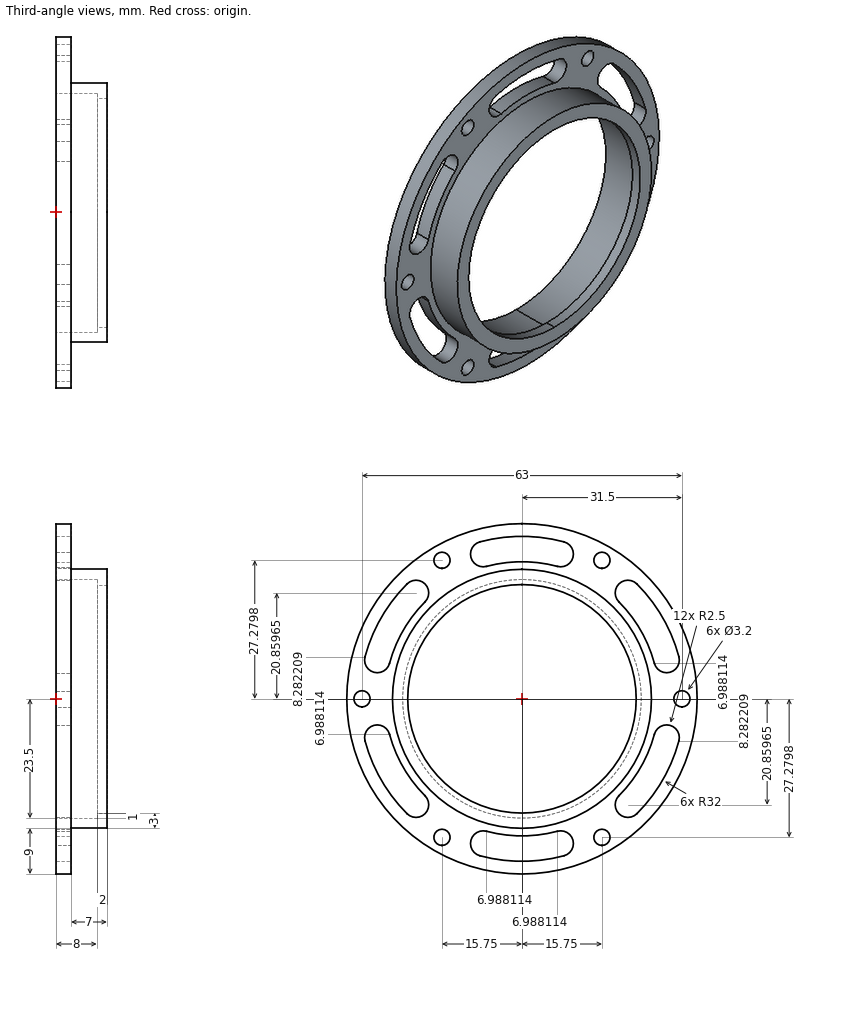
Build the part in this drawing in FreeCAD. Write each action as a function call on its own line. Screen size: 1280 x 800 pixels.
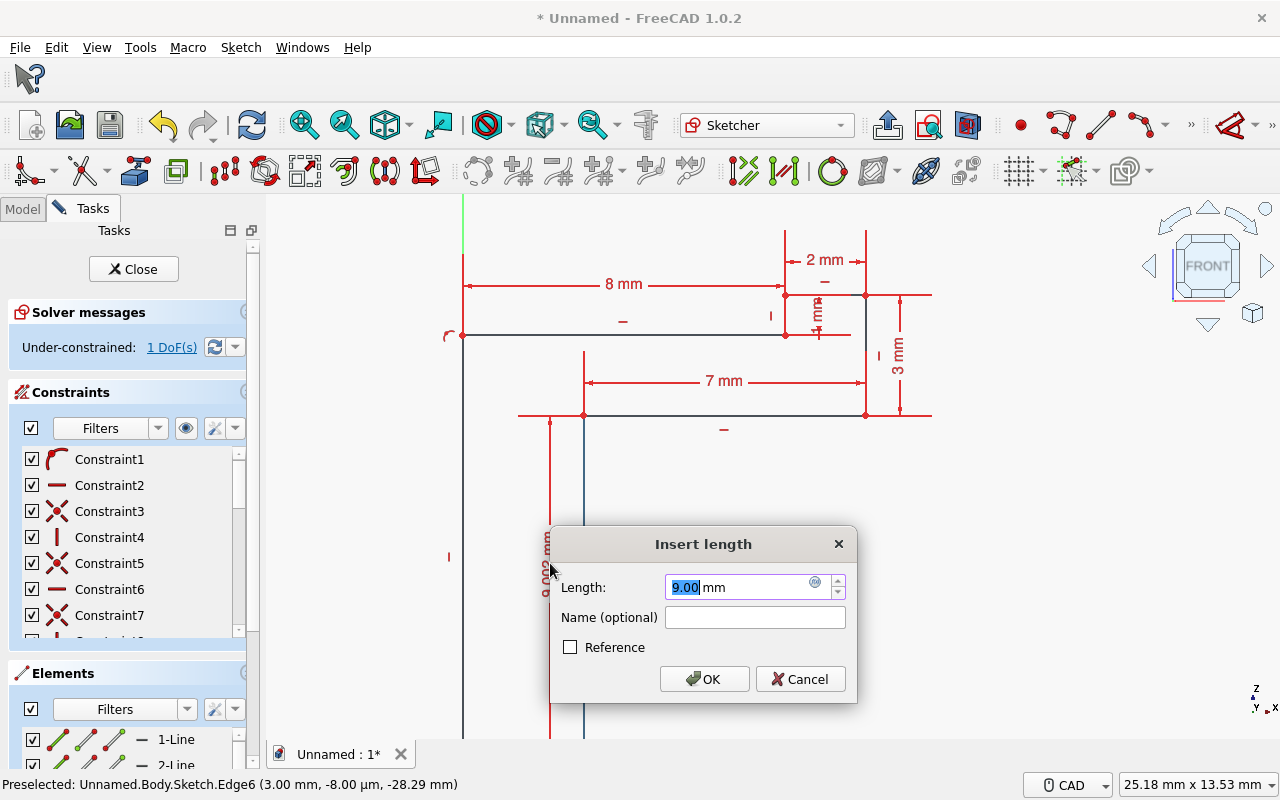
text(9)
key(Return)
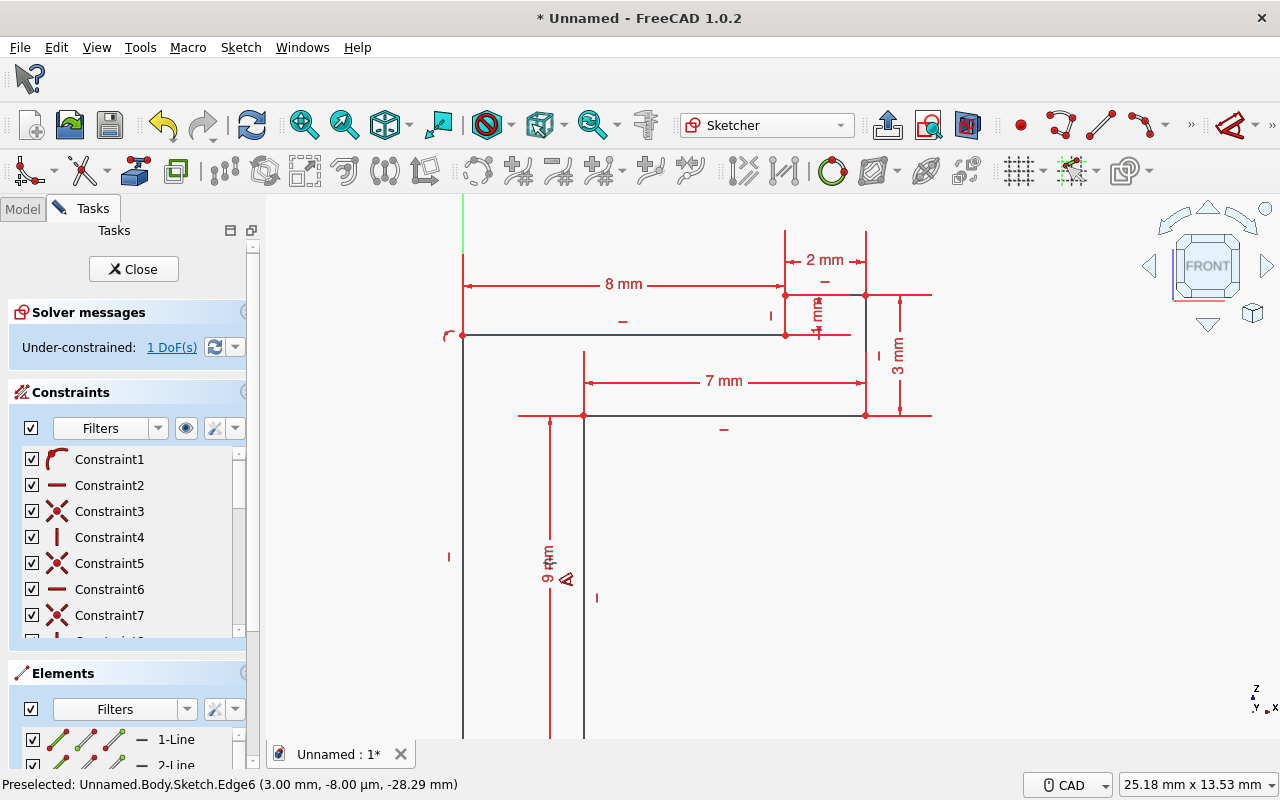
click(463, 335)
click(429, 279)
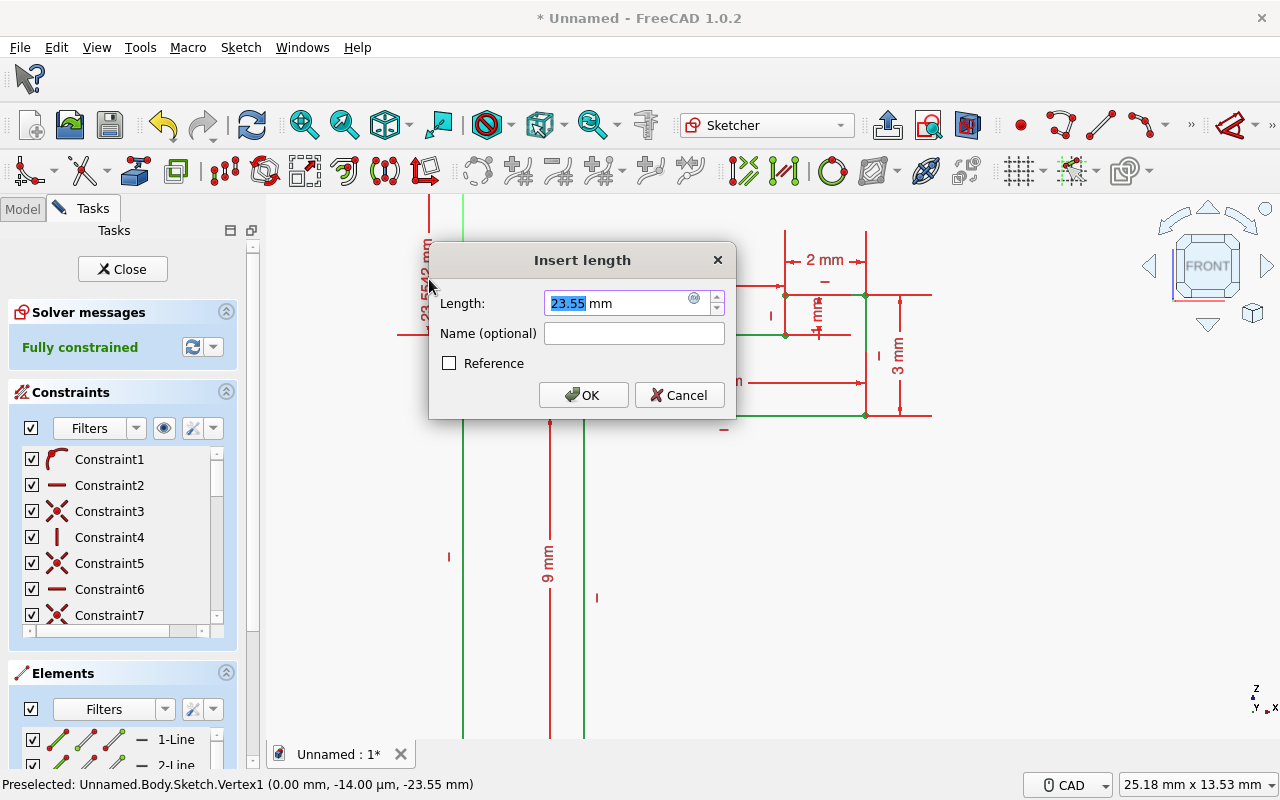
text(23.5)
key(Return)
key(Escape)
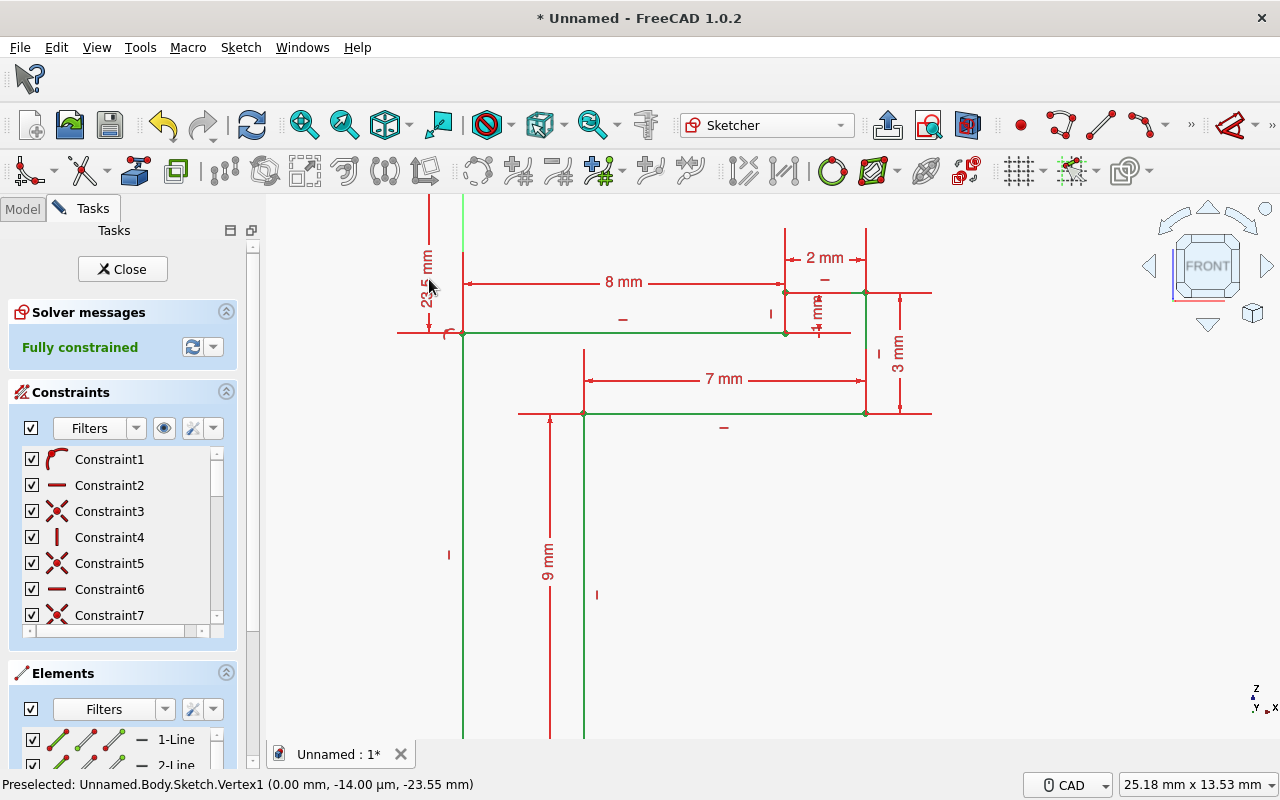
click(123, 269)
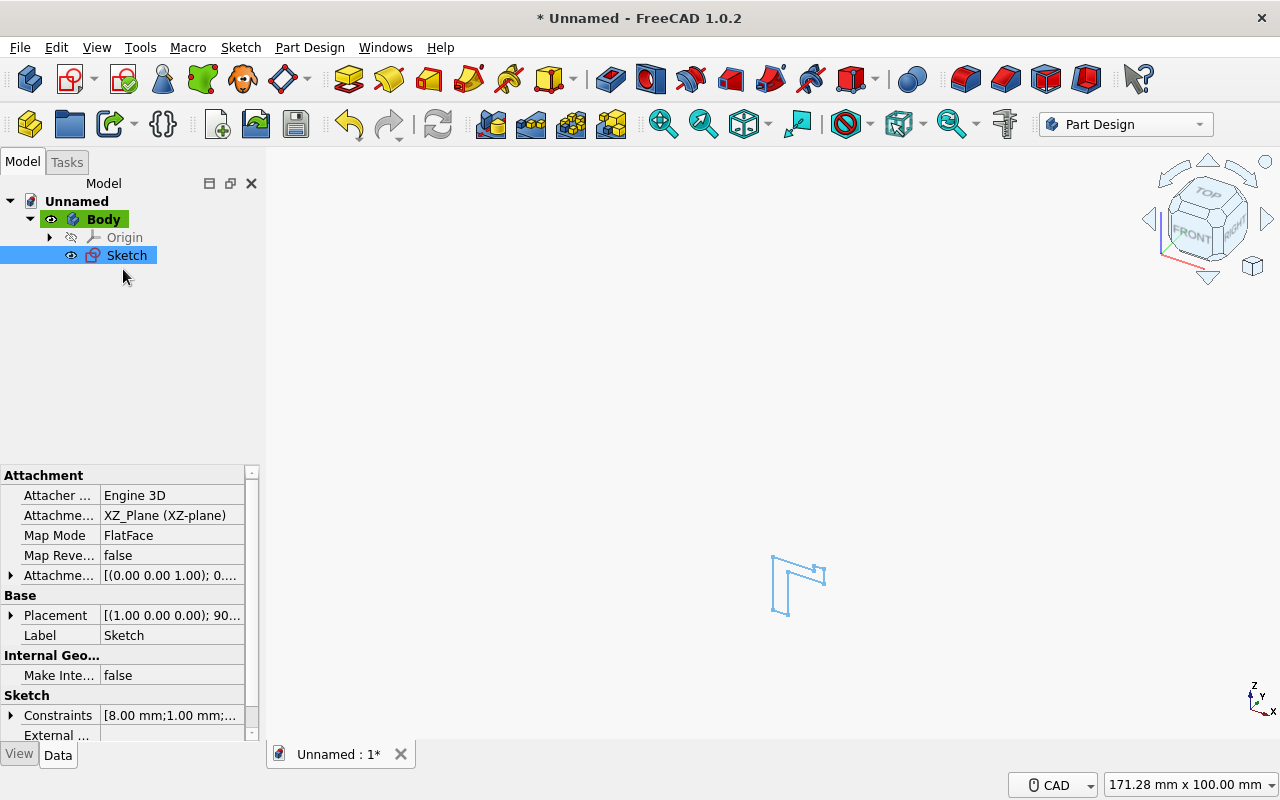
click(390, 80)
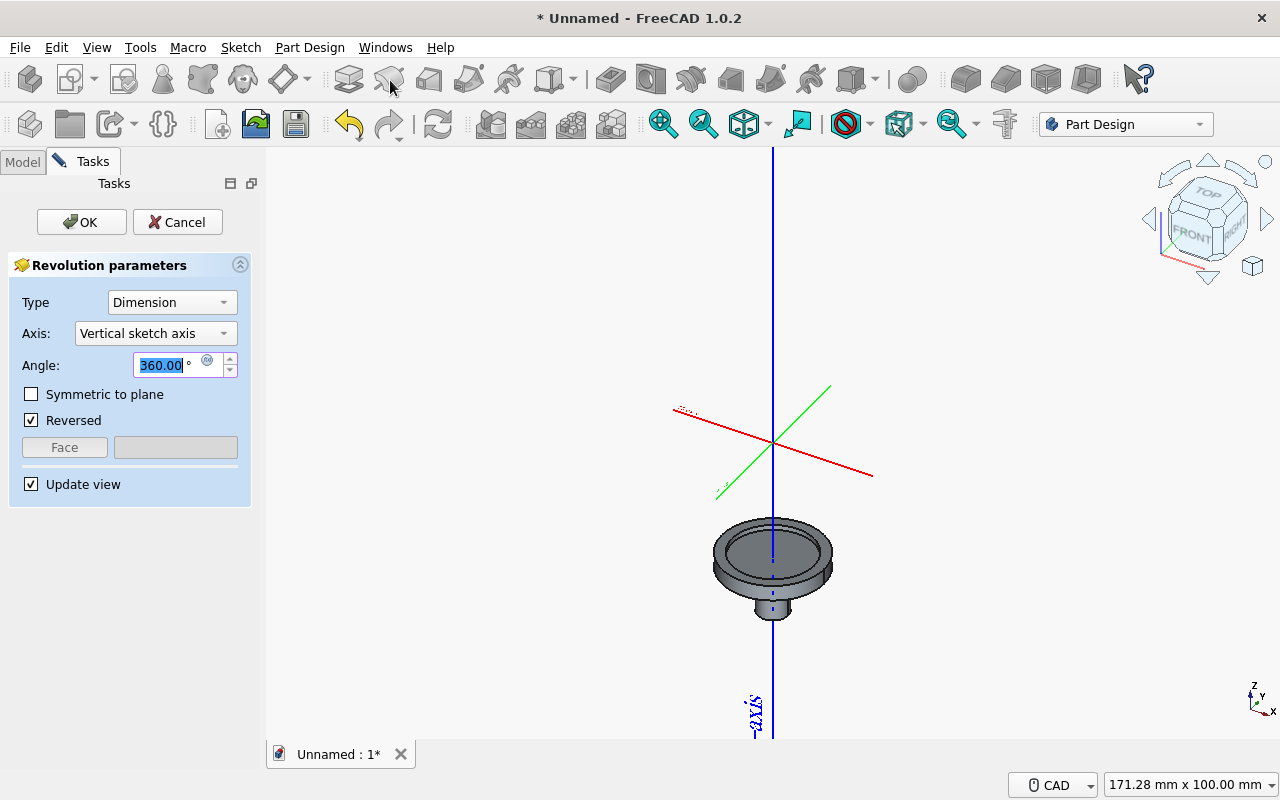
click(156, 334)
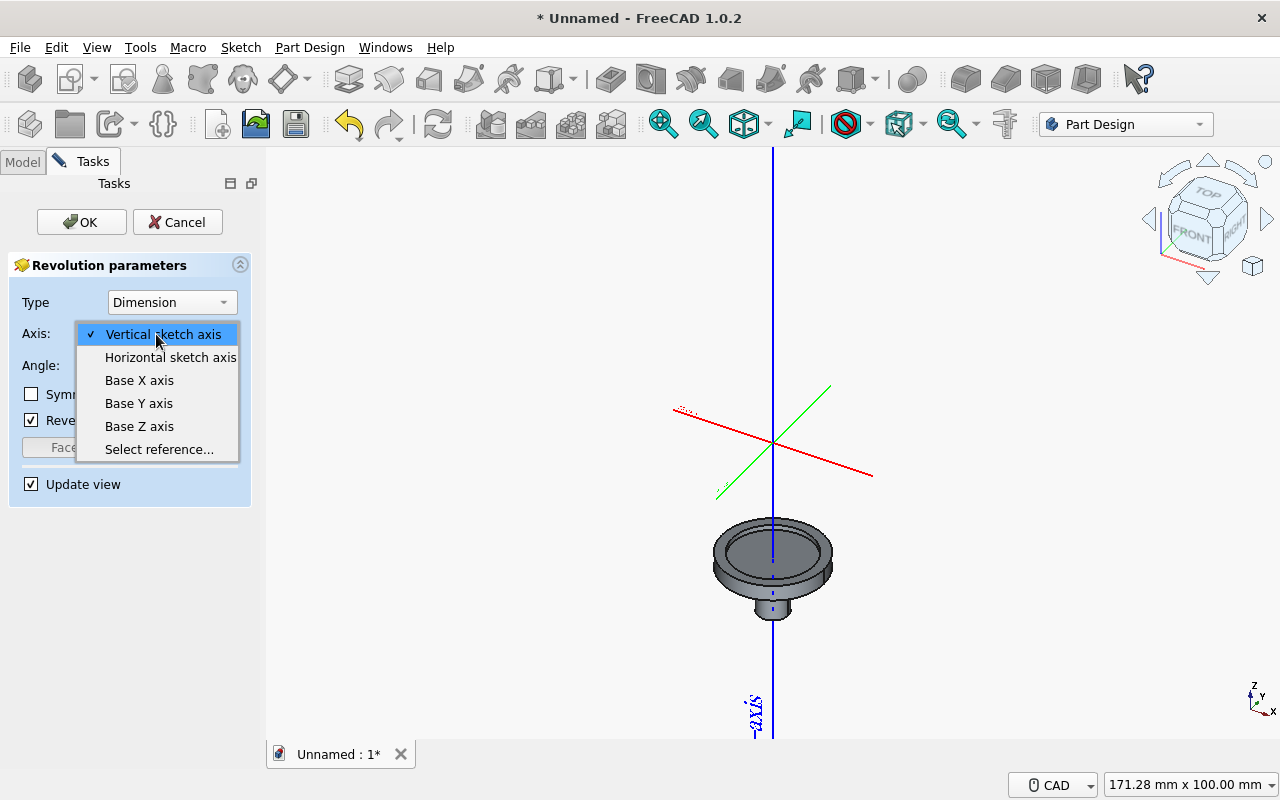
click(156, 358)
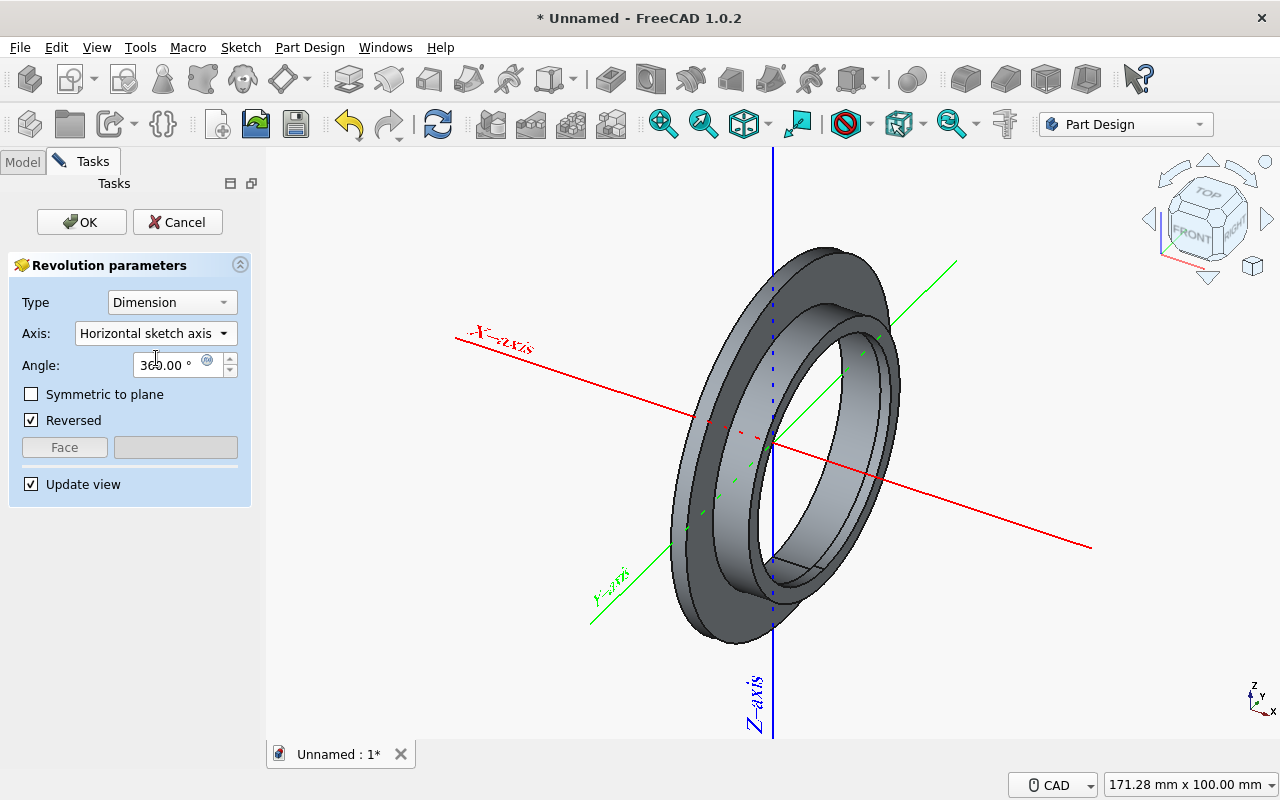
click(82, 222)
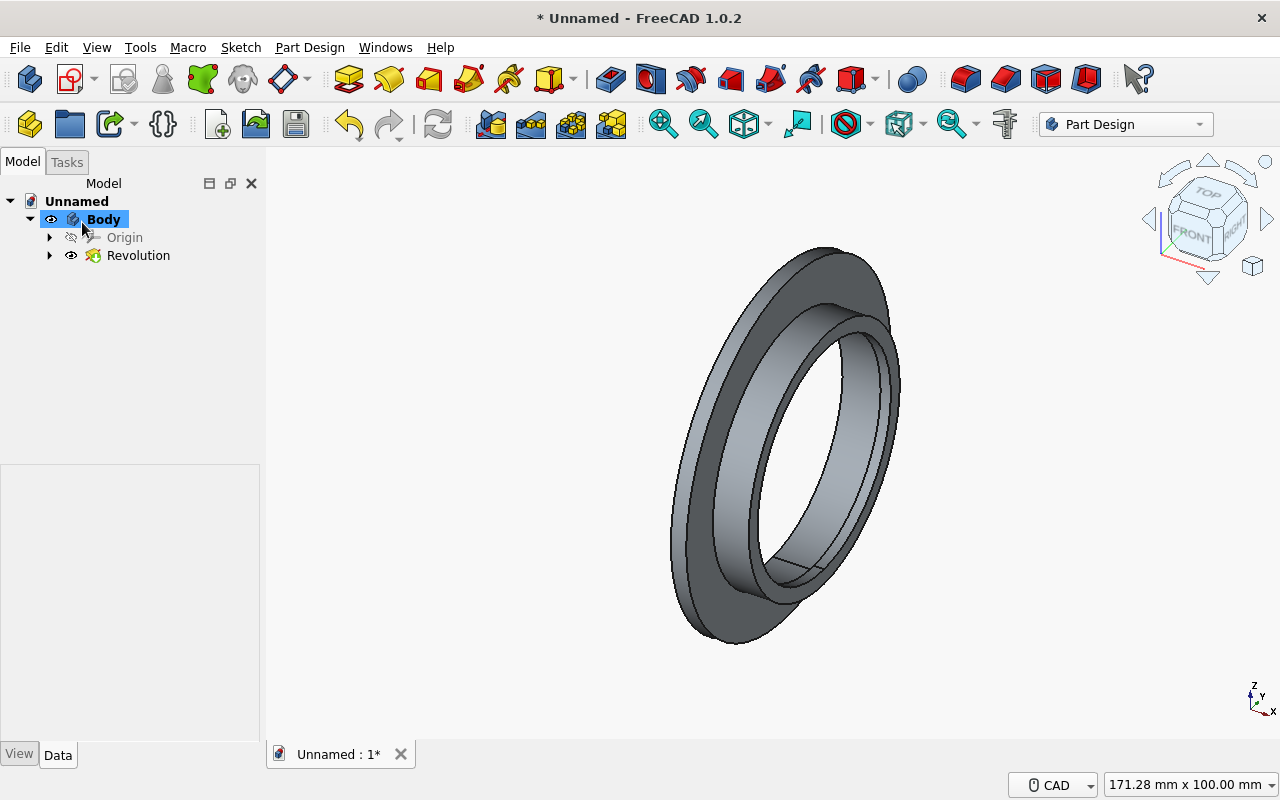
click(788, 304)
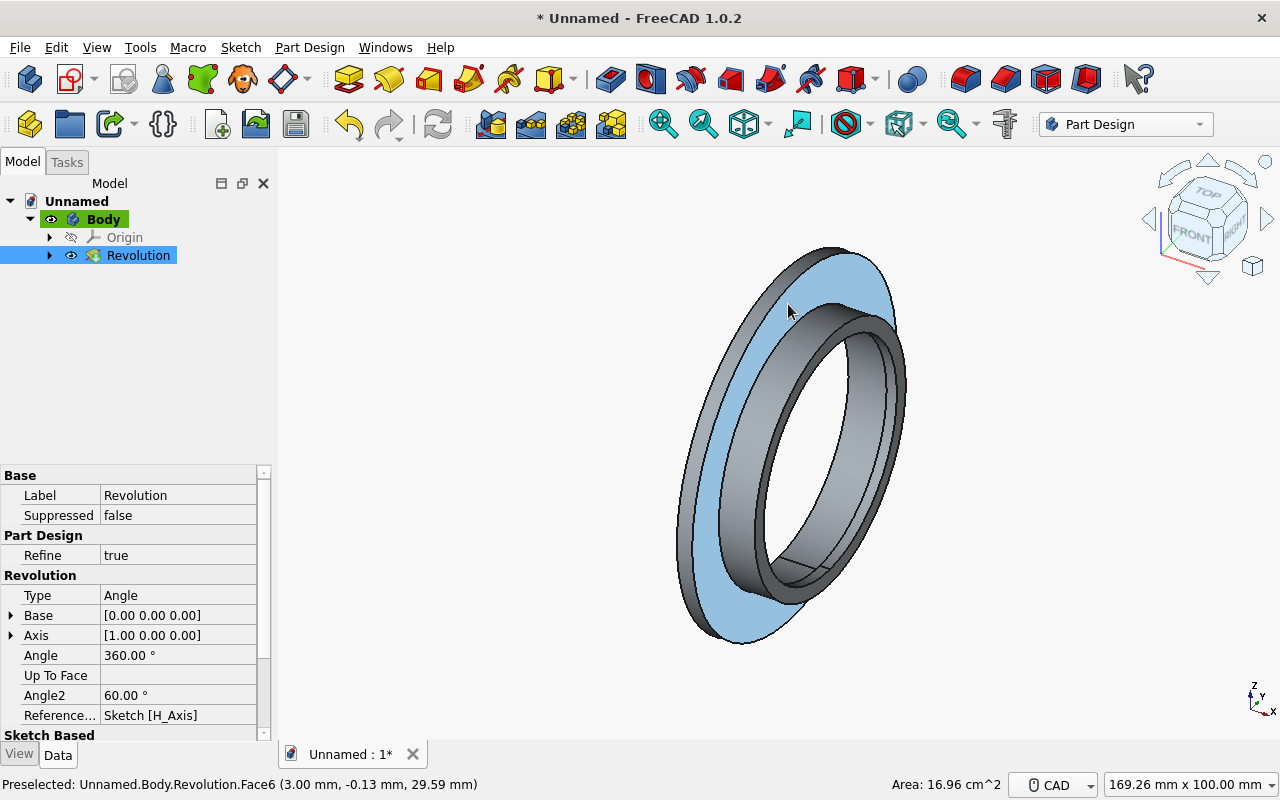
click(70, 80)